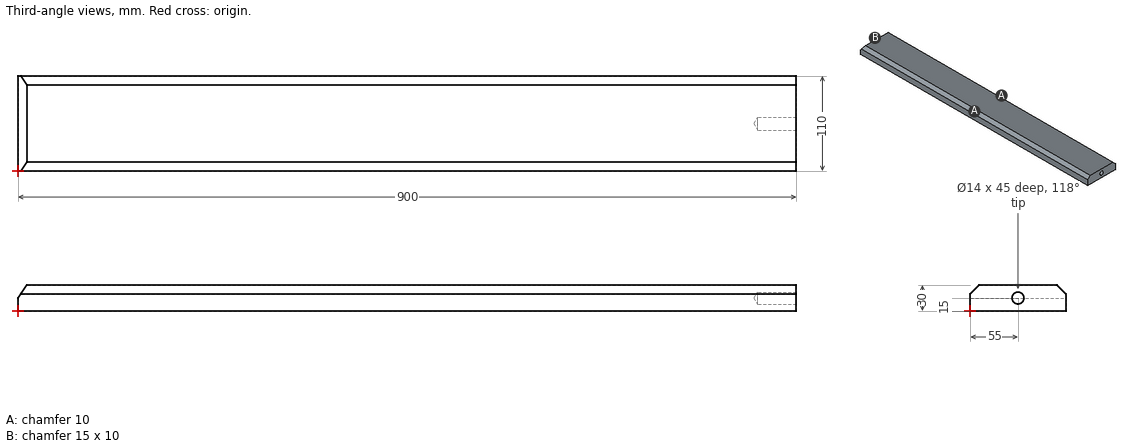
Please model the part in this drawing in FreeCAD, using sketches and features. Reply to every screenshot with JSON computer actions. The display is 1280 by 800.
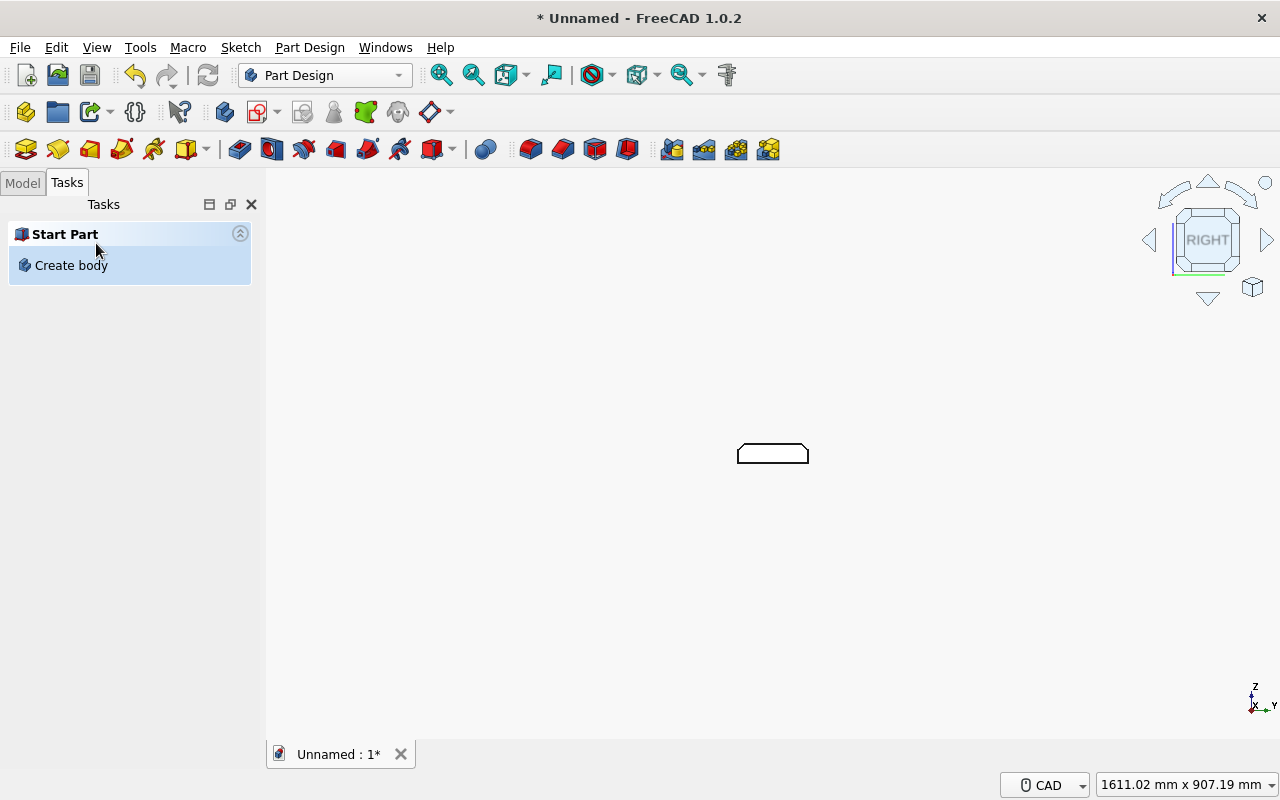
{"action": "key", "text": "v f"}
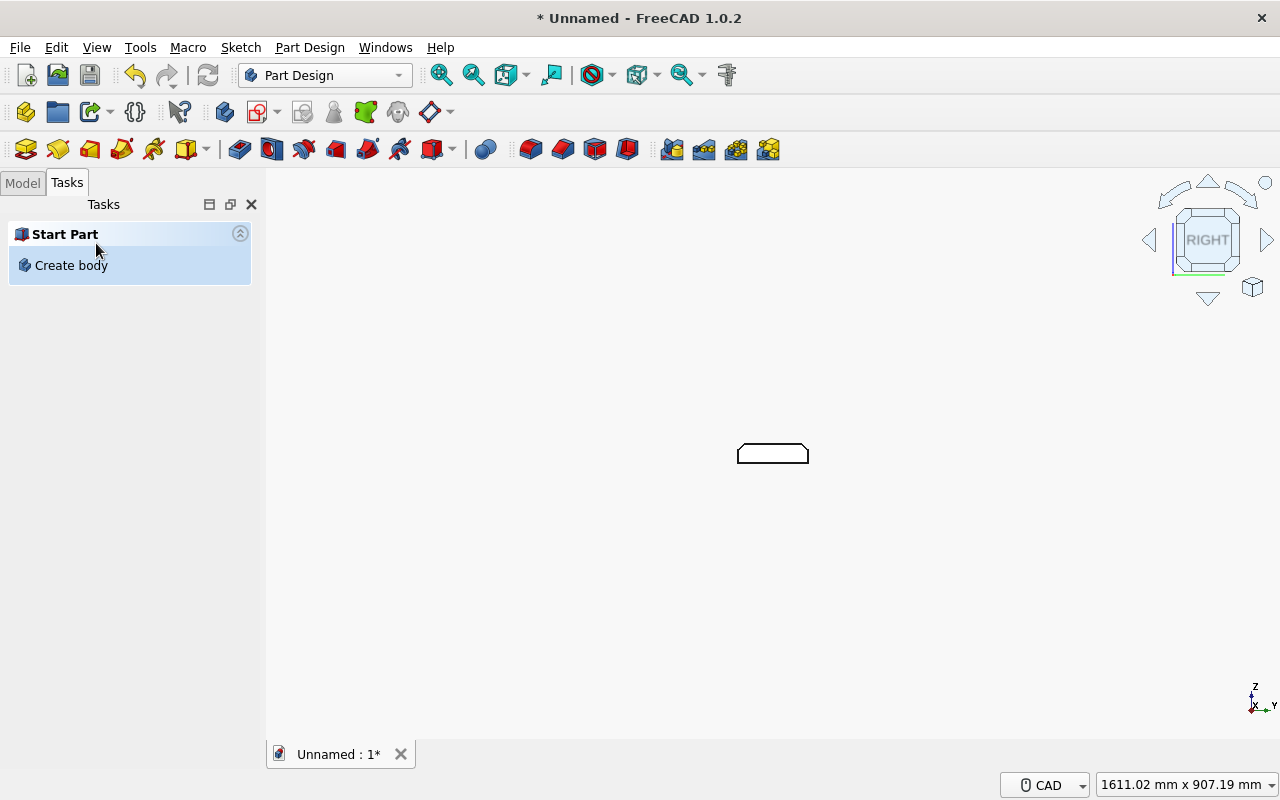
{"action": "left_click", "coordinate": [793, 452]}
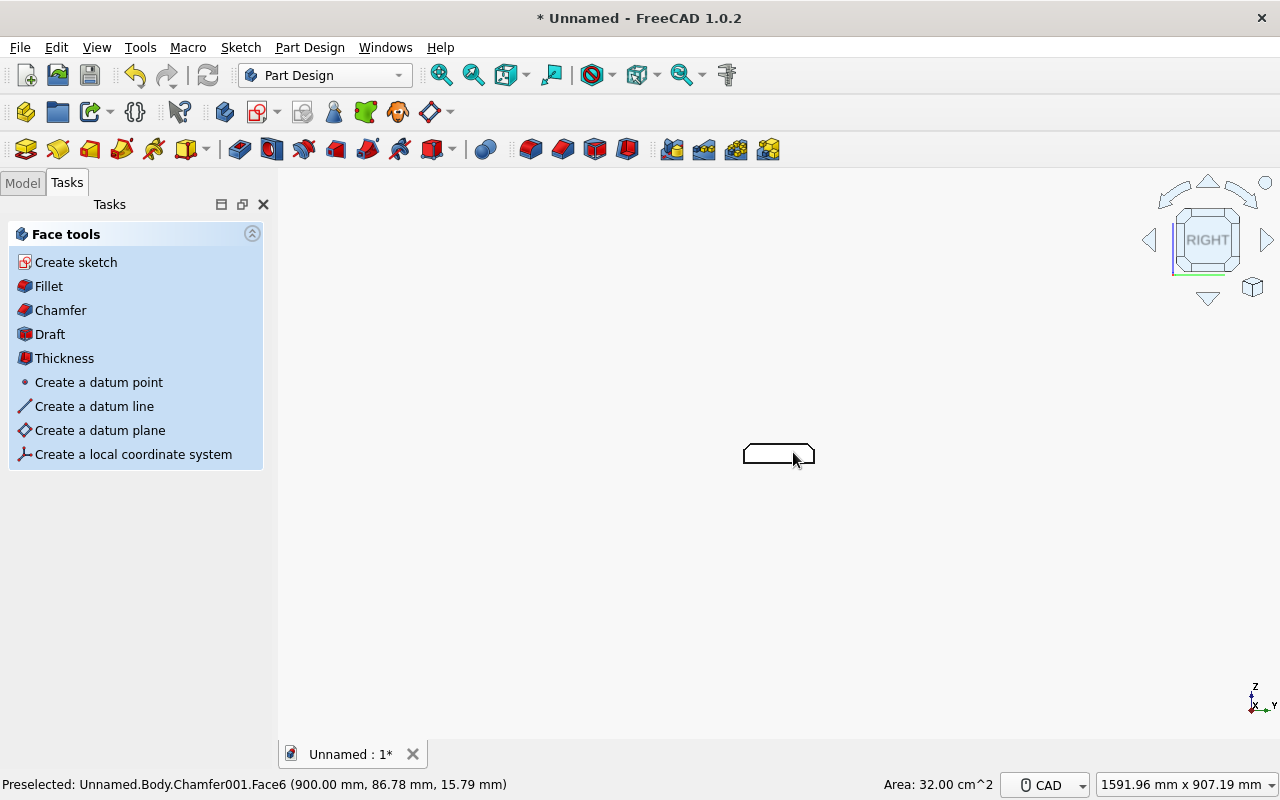
{"action": "left_click", "coordinate": [258, 112]}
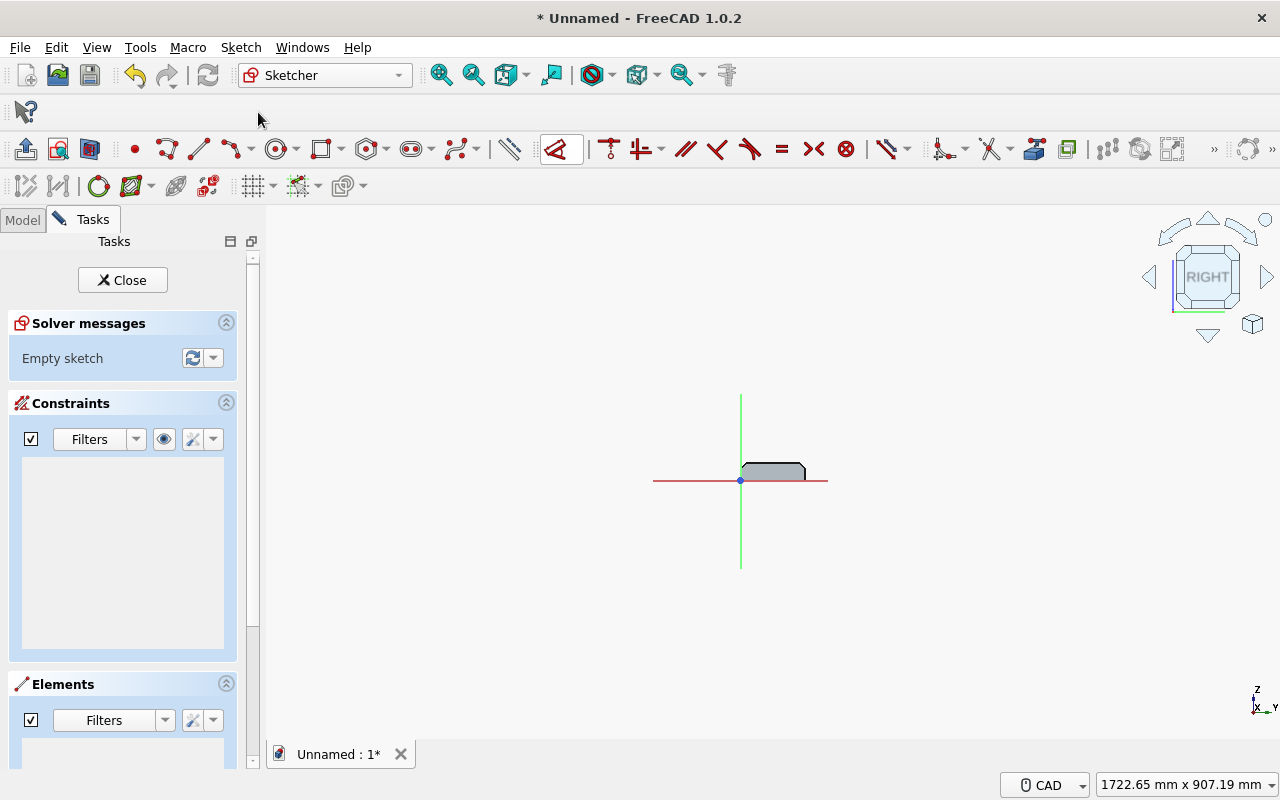
{"action": "scroll", "coordinate": [777, 472], "scroll_direction": "up", "scroll_amount": 15}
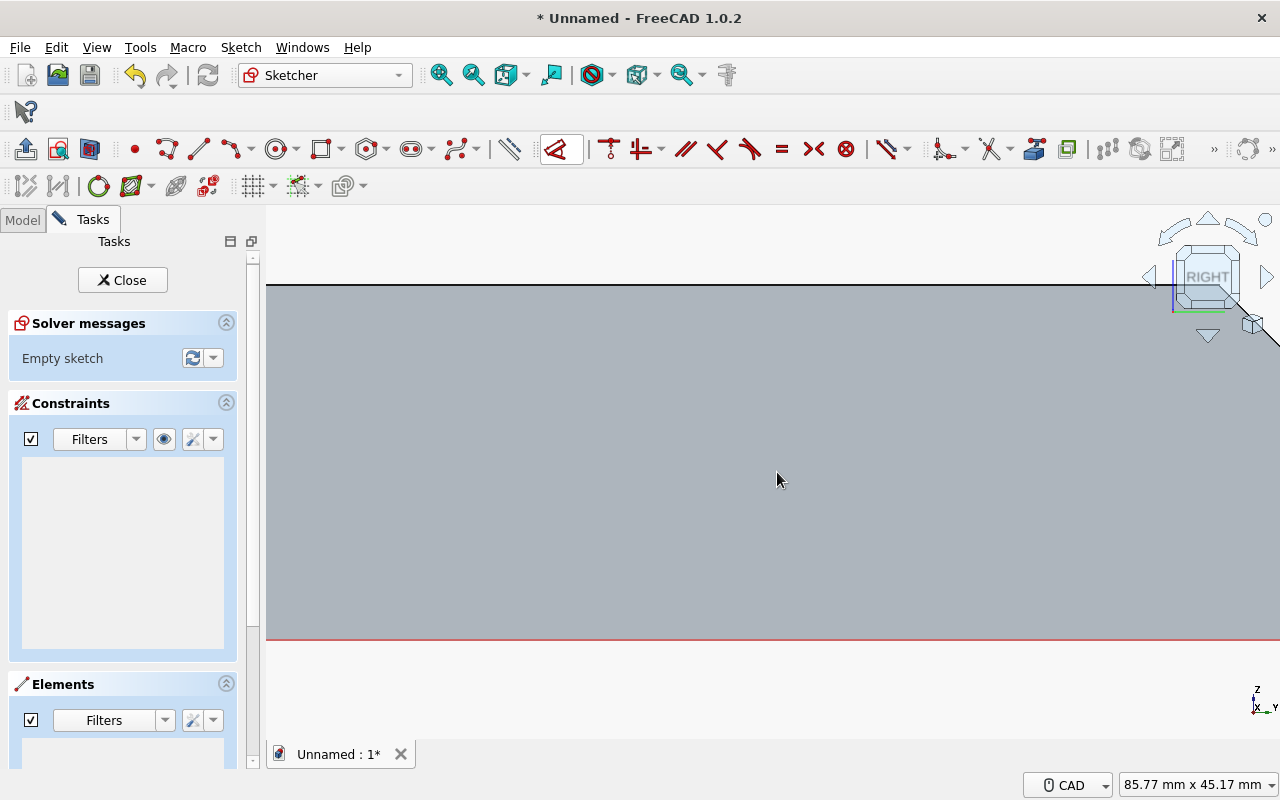
{"action": "scroll", "coordinate": [673, 455], "scroll_direction": "up", "scroll_amount": 4}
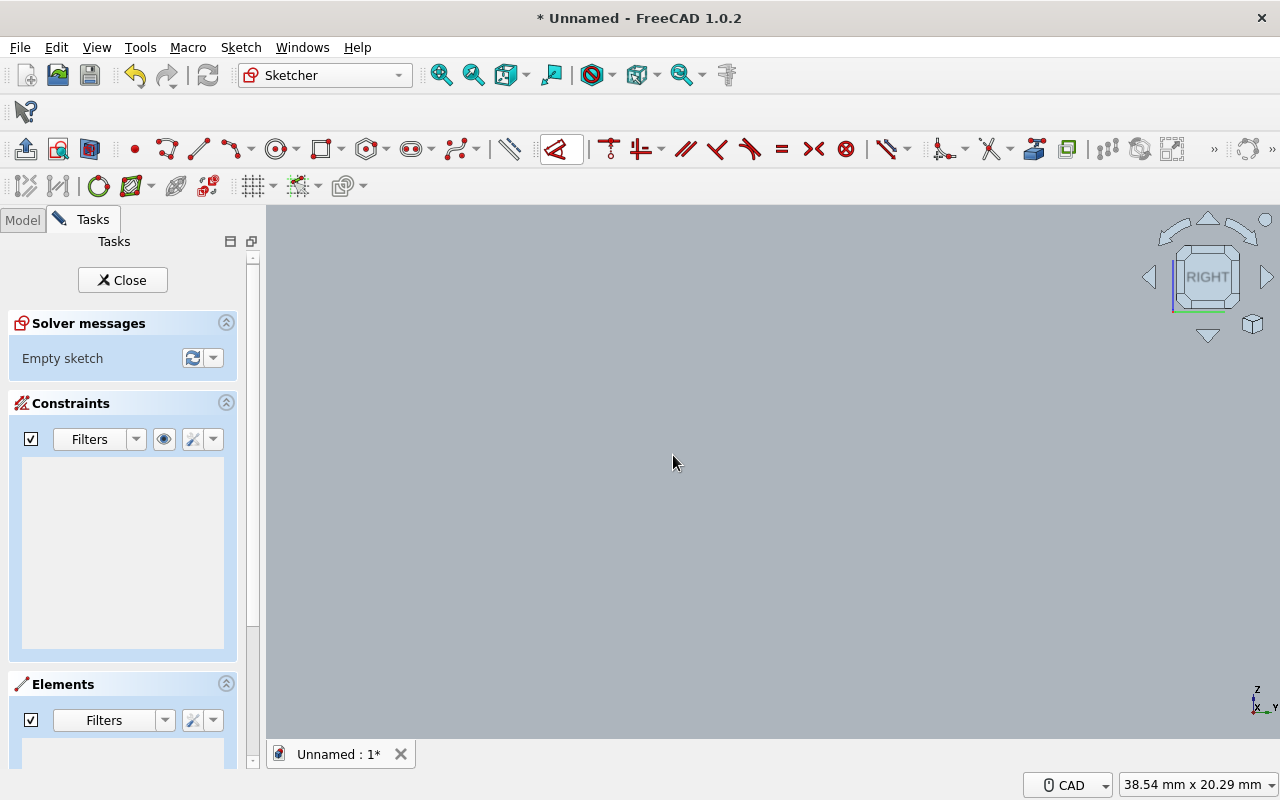
{"action": "key", "text": "g c"}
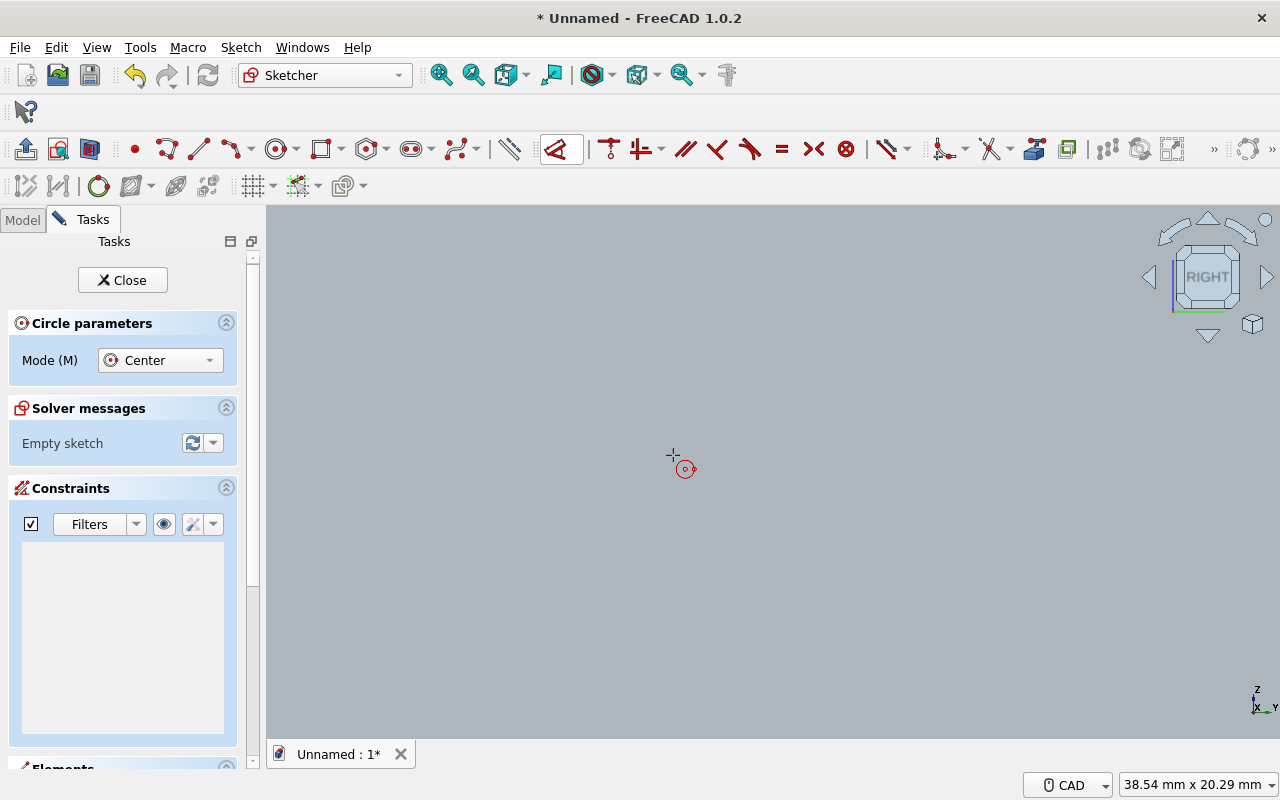
{"action": "left_click", "coordinate": [704, 471]}
{"action": "mouse_move", "coordinate": [834, 341]}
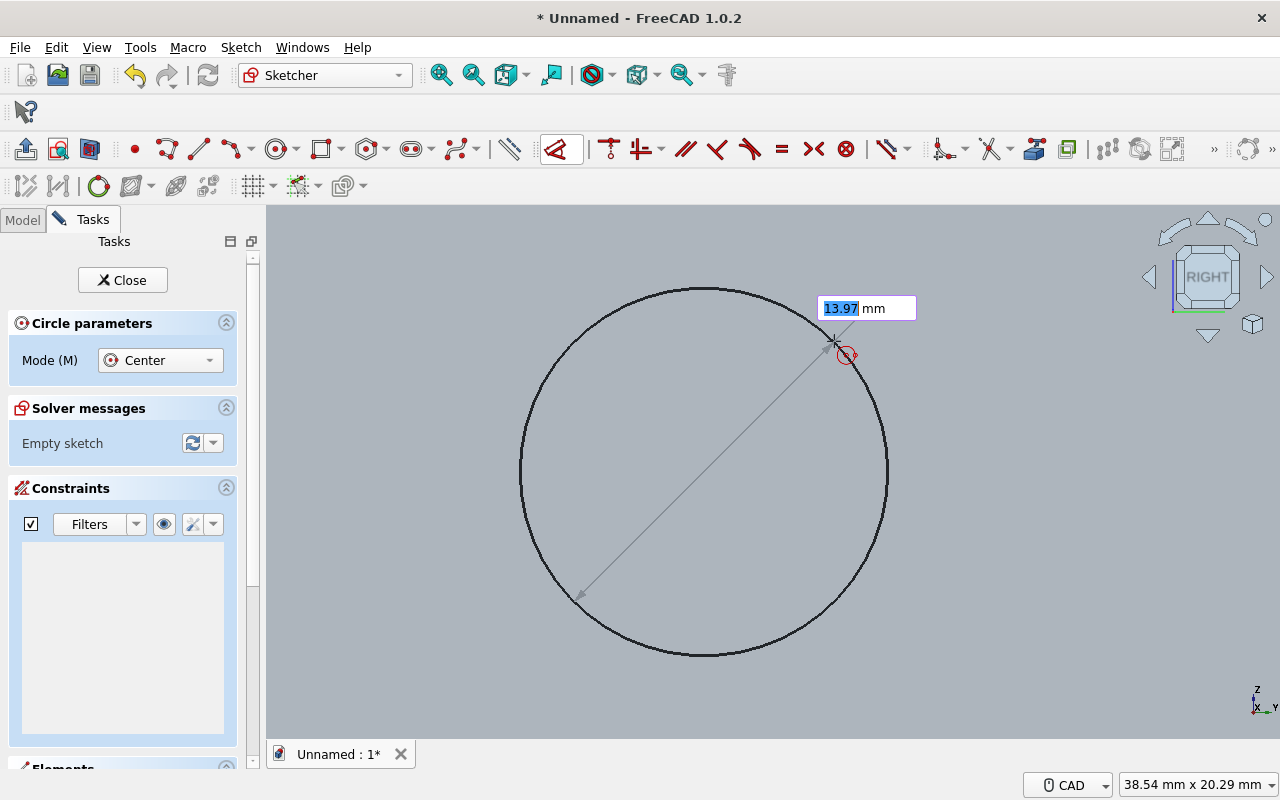
{"action": "type", "text": "14"}
{"action": "key", "text": "Return"}
{"action": "key", "text": "Escape"}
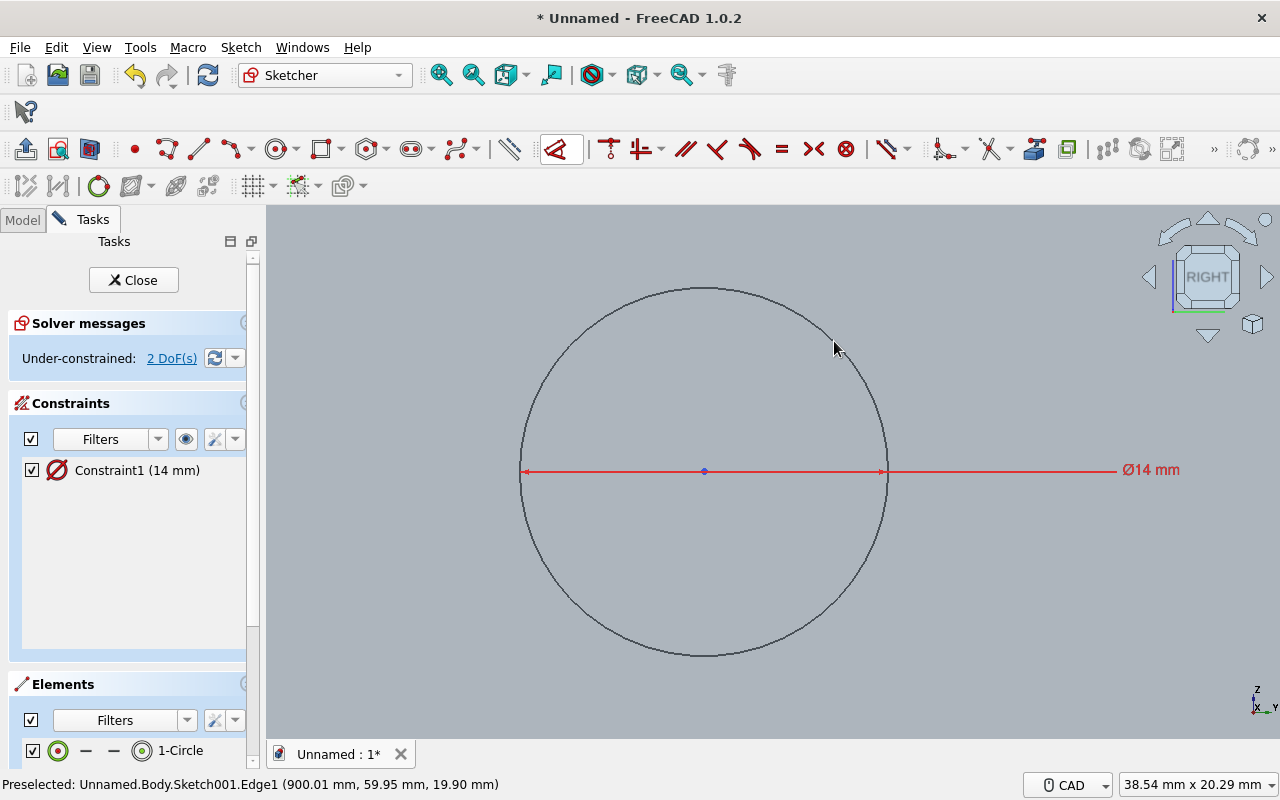
{"action": "key", "text": "d"}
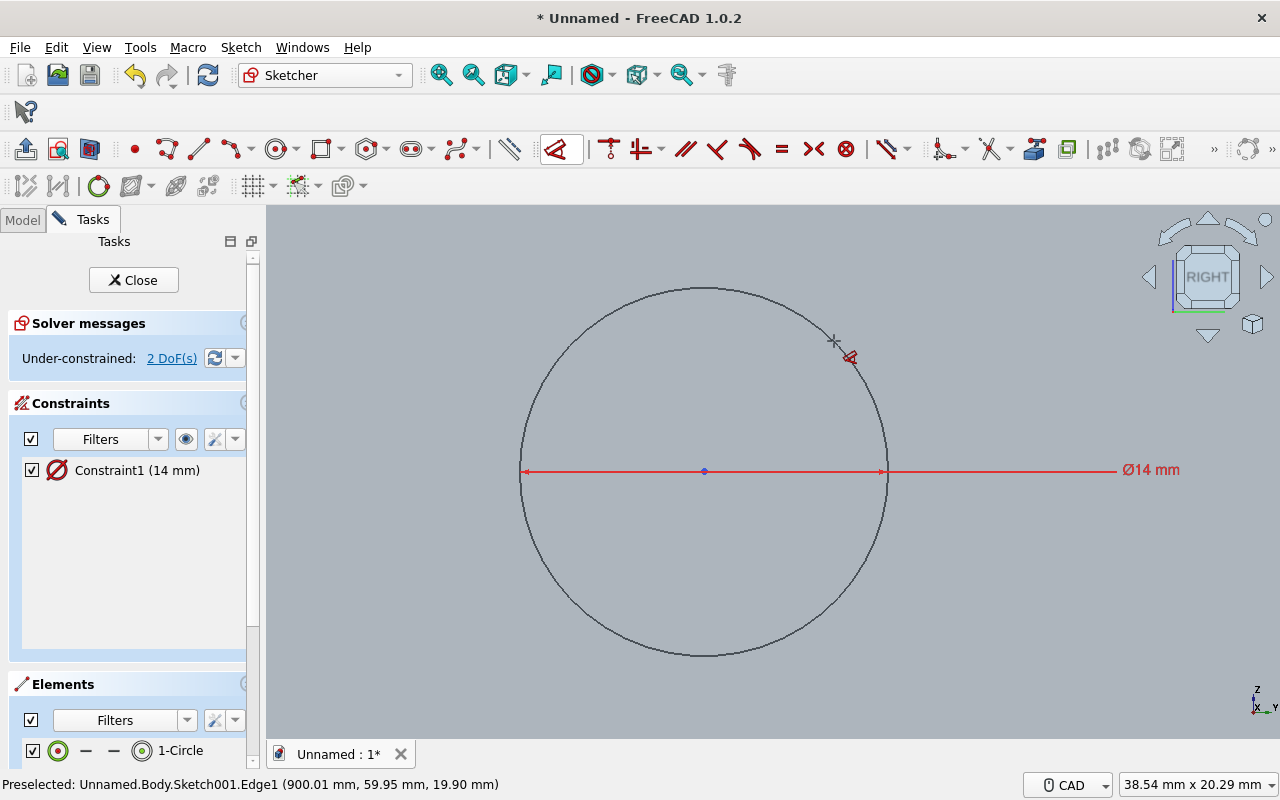
{"action": "left_click", "coordinate": [704, 472]}
{"action": "left_click", "coordinate": [499, 438]}